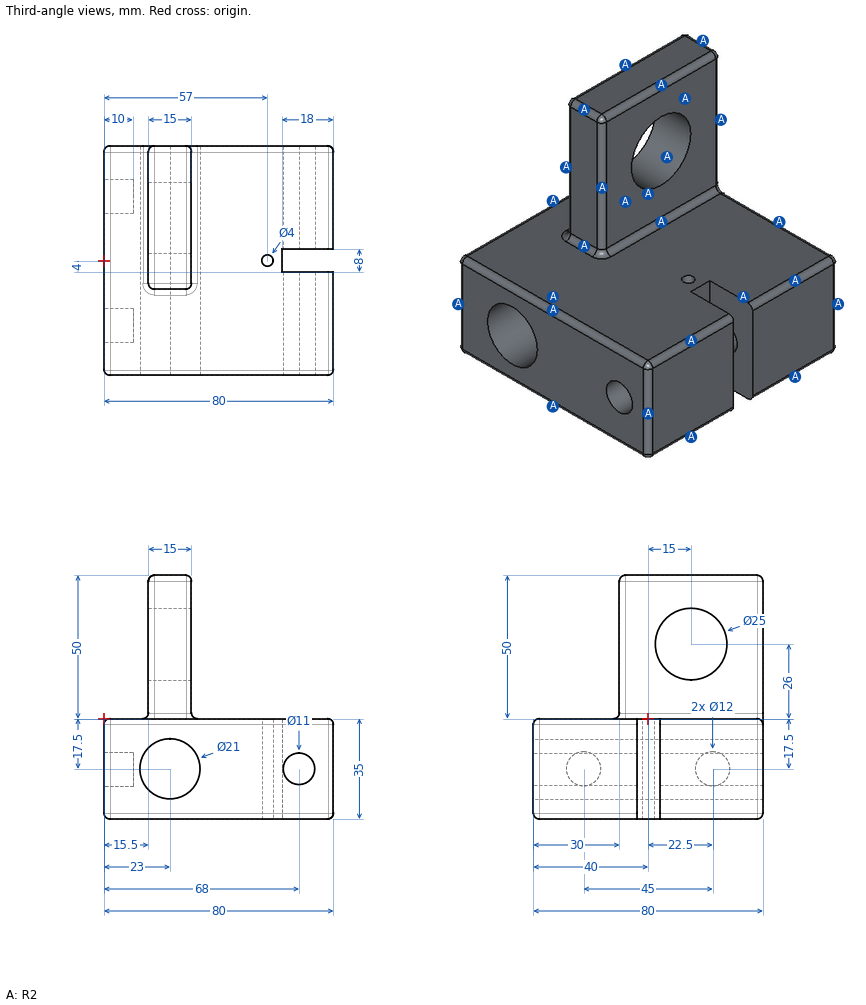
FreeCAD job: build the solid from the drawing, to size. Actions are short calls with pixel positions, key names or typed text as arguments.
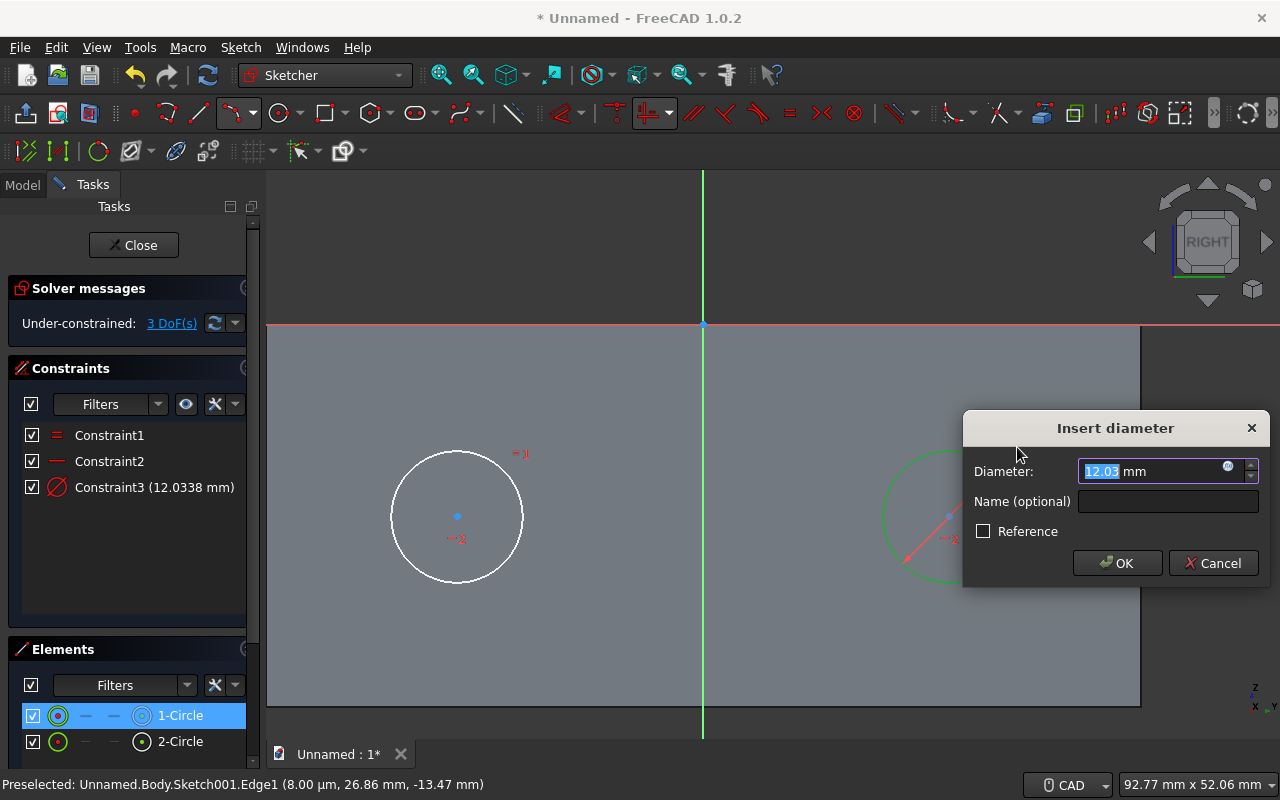
text(12)
key(Return)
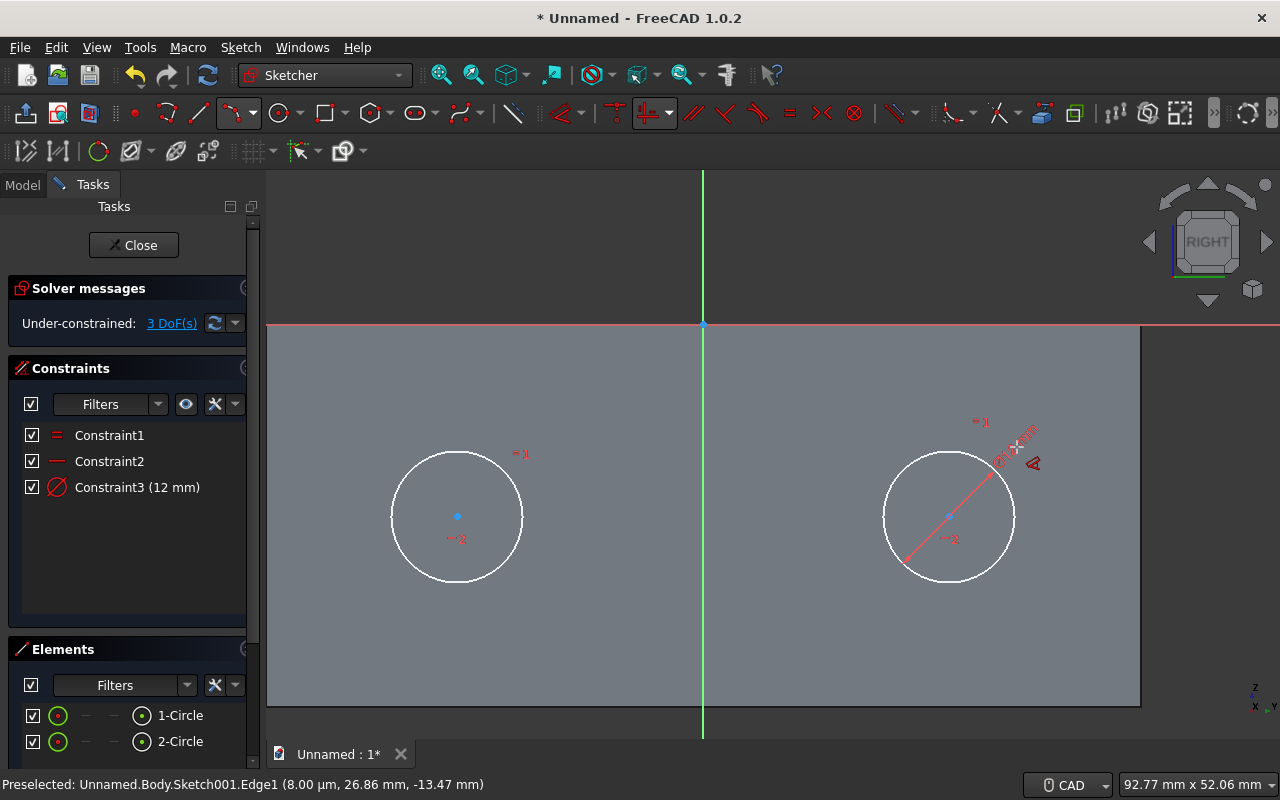
click(949, 517)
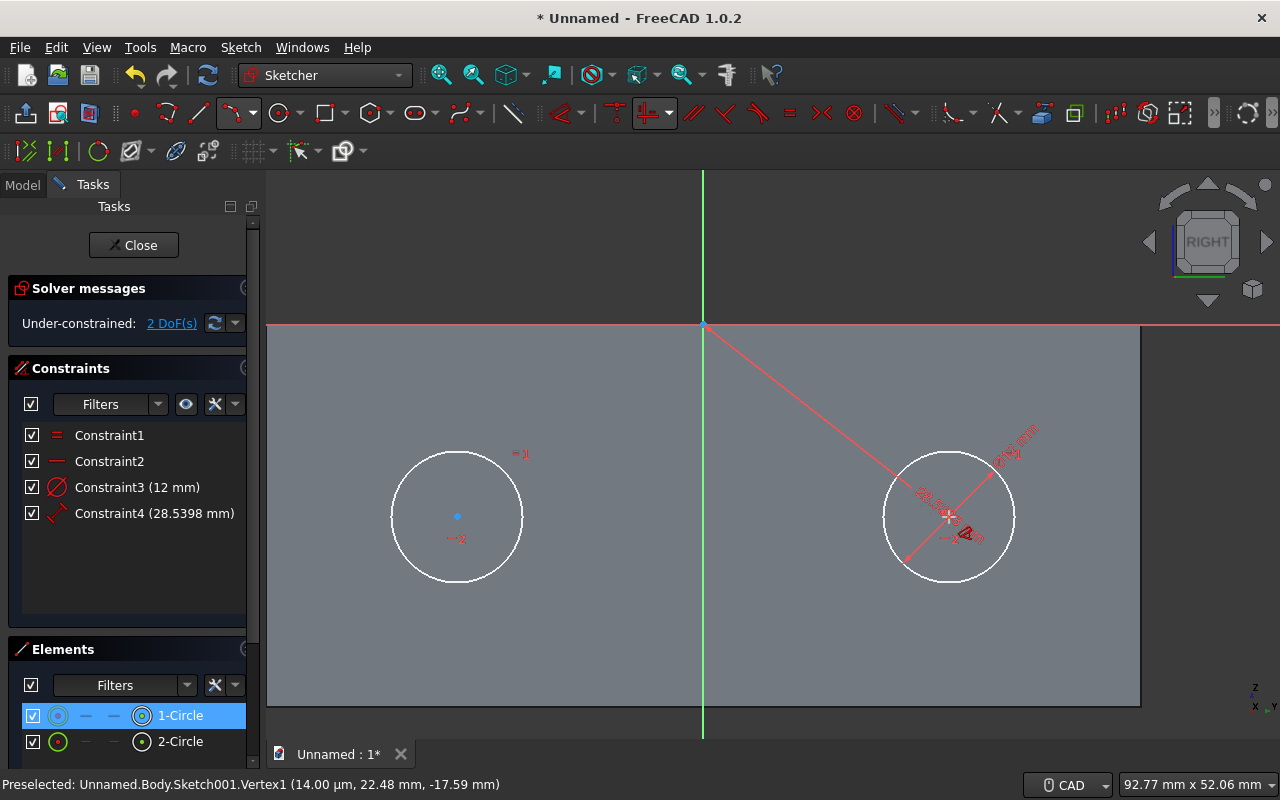
click(457, 517)
click(590, 551)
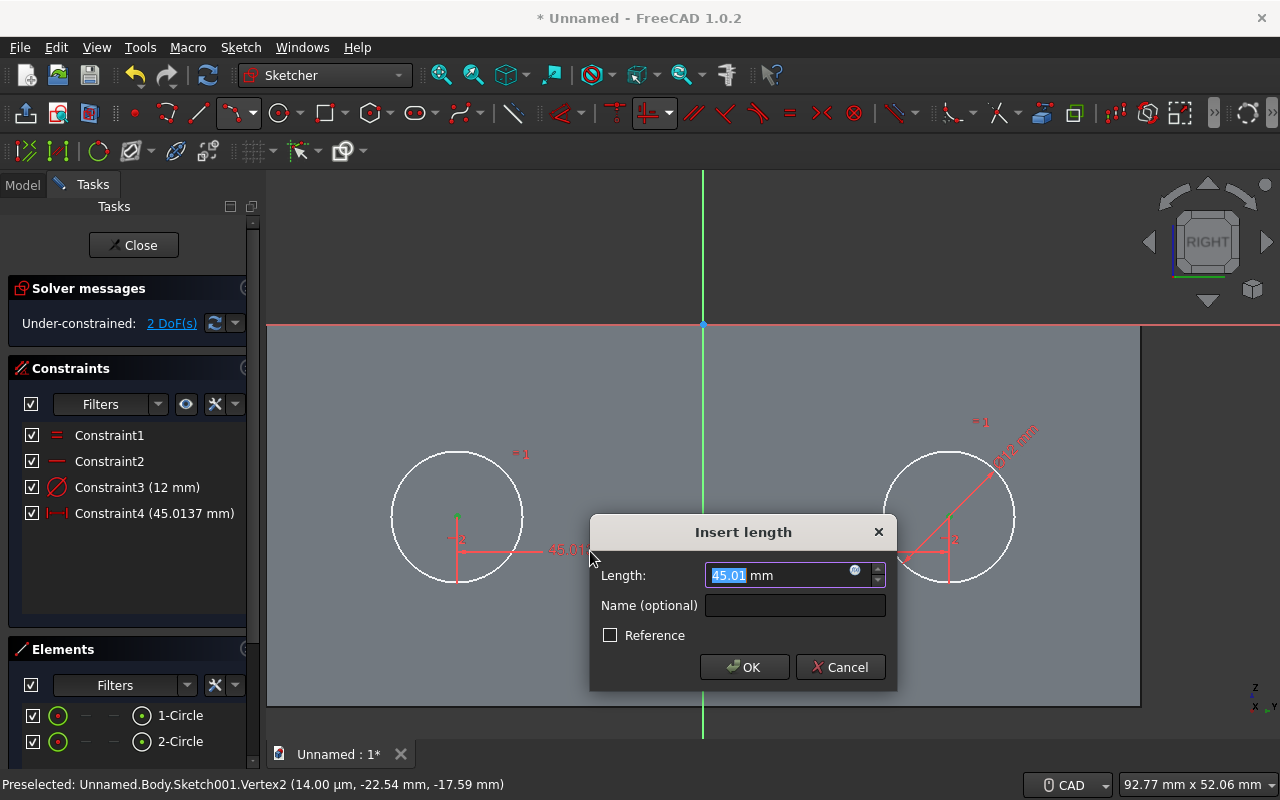
text(45)
key(Return)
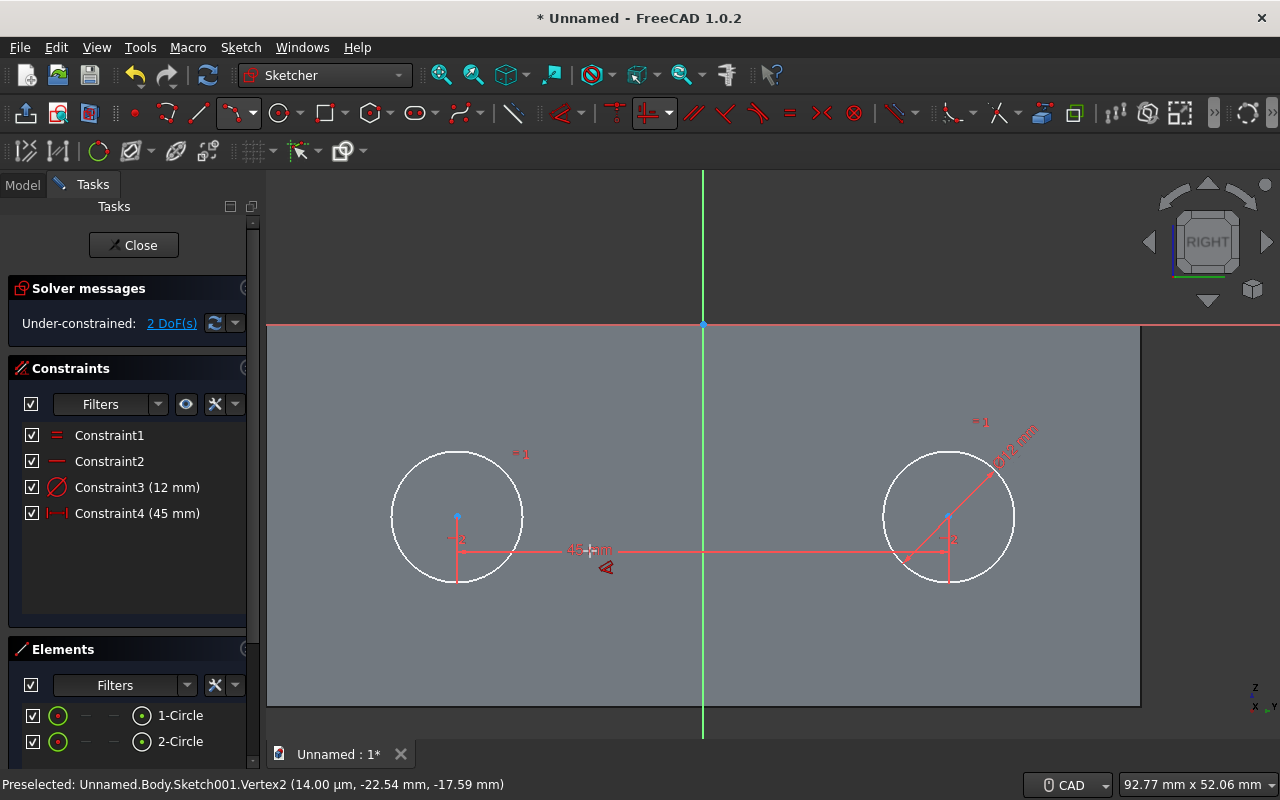
click(949, 517)
click(826, 291)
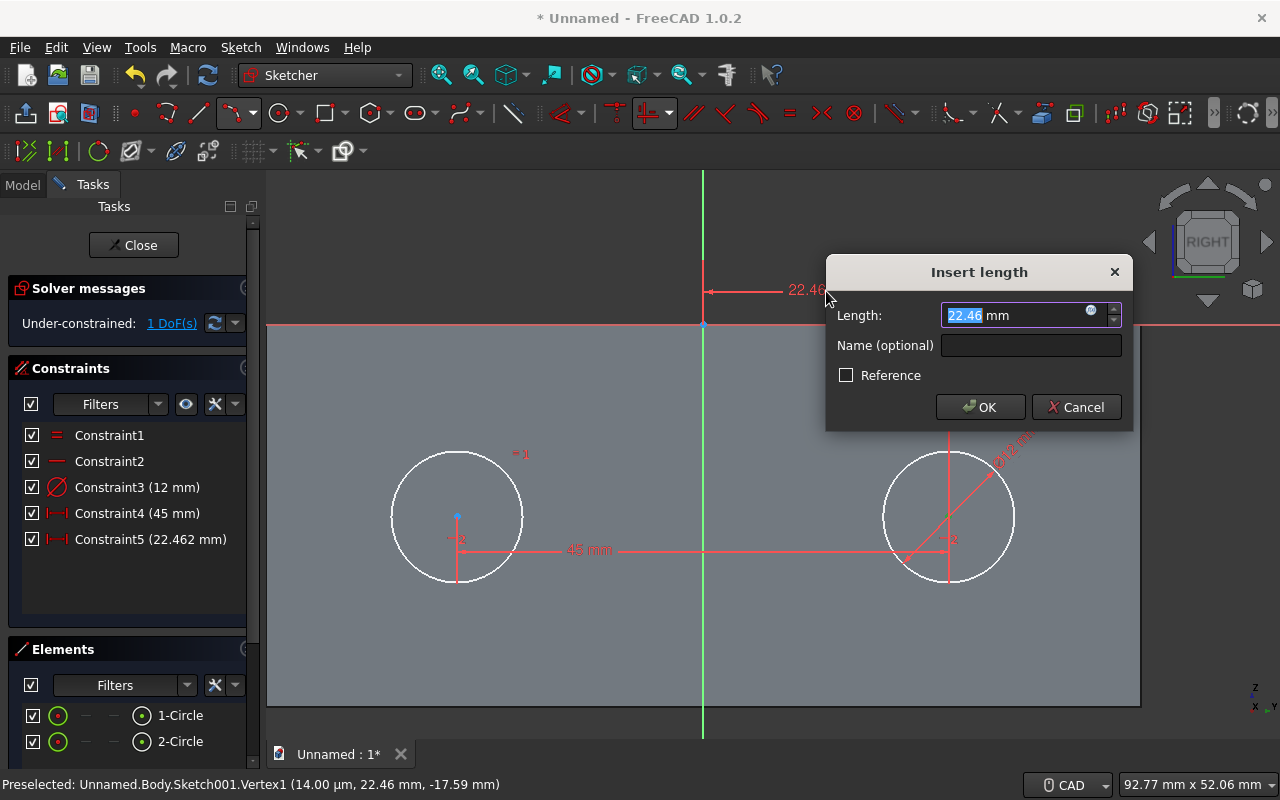
text(22.5)
key(Return)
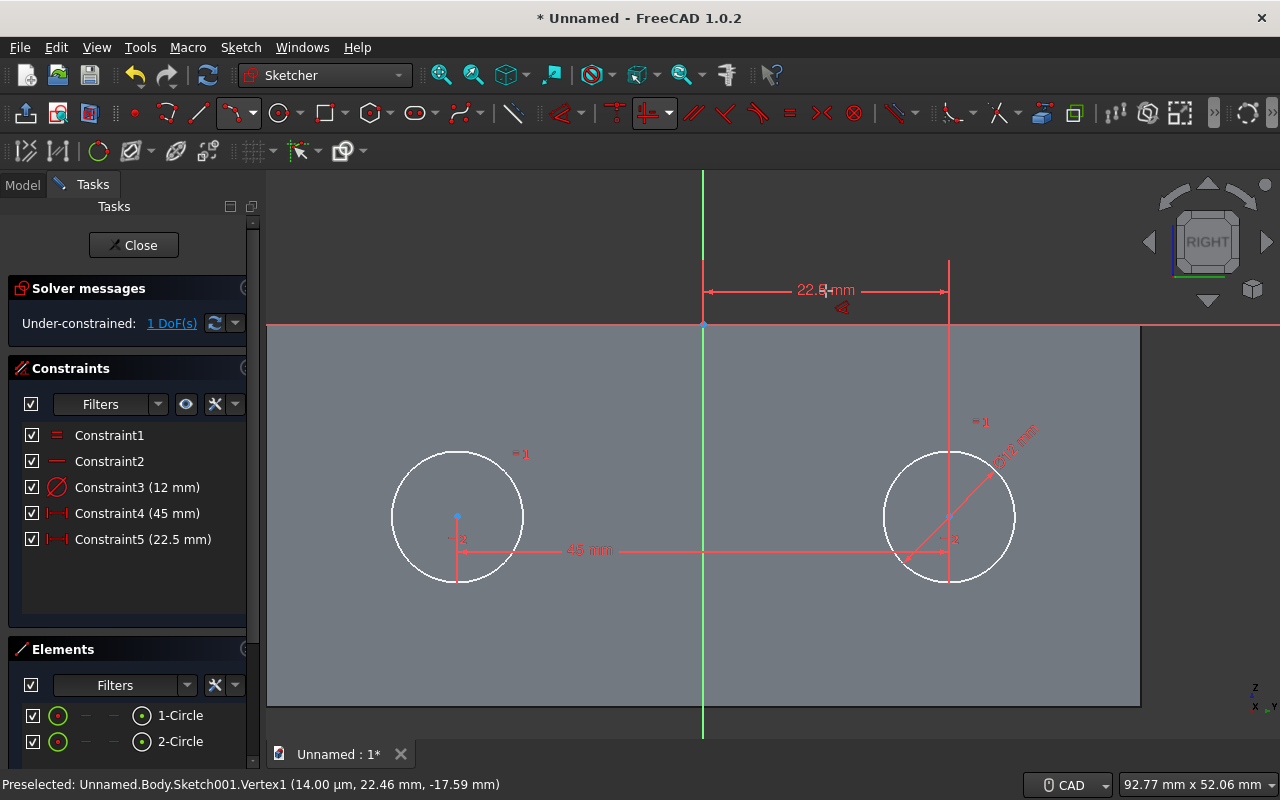
click(949, 517)
click(983, 421)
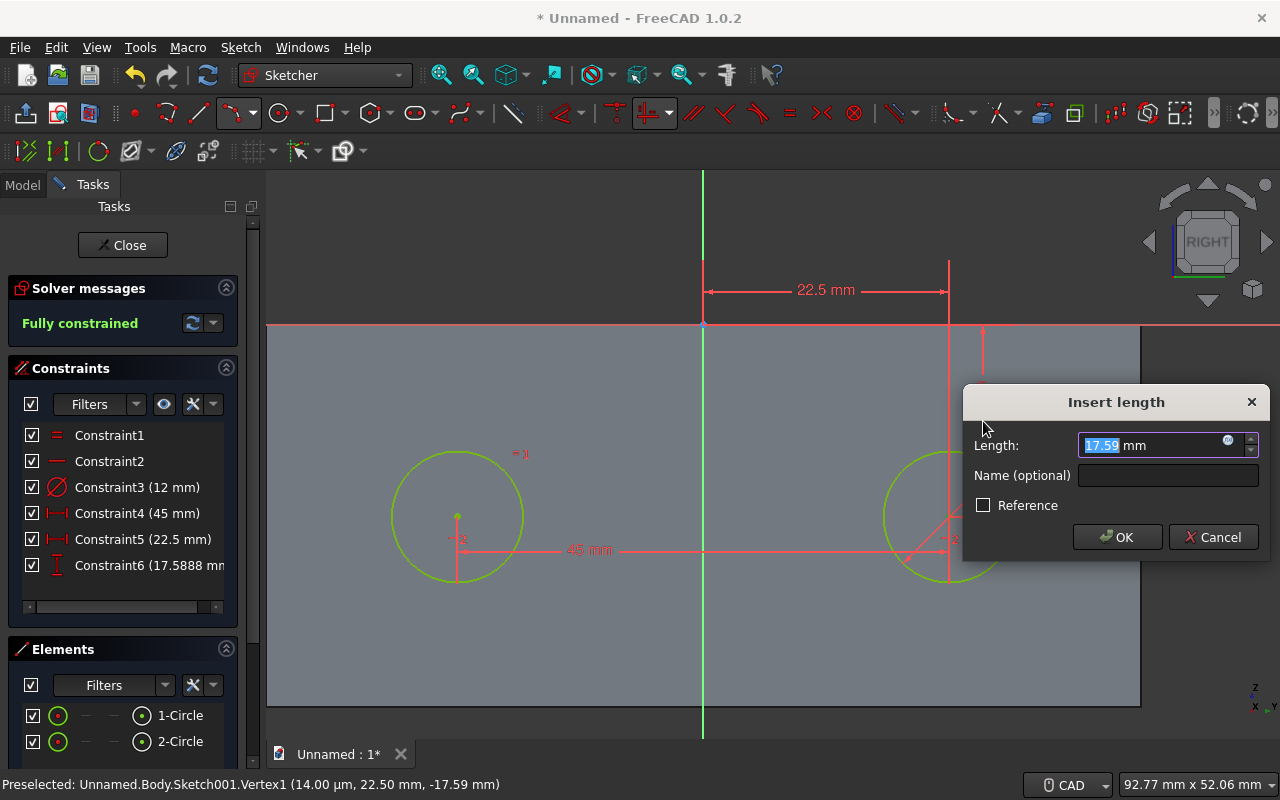
text(17.5)
key(Return)
key(Escape)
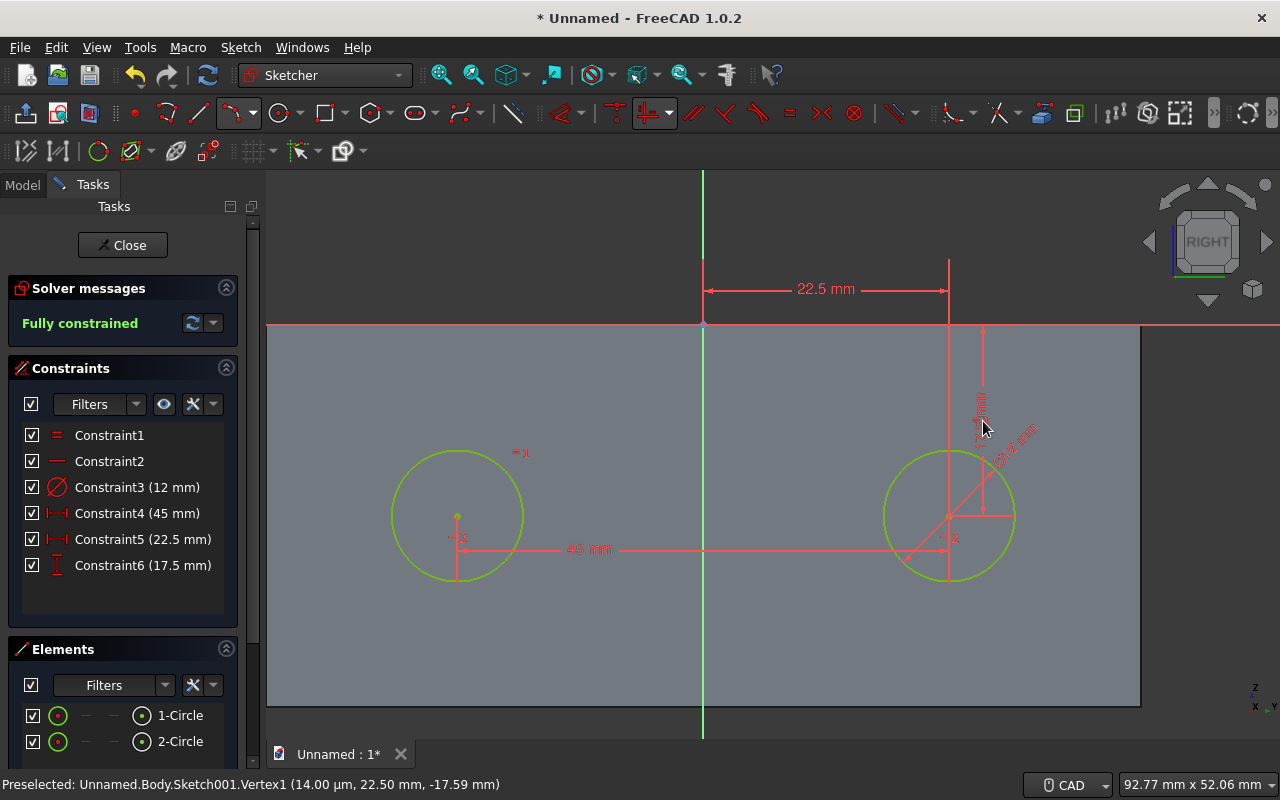
click(123, 245)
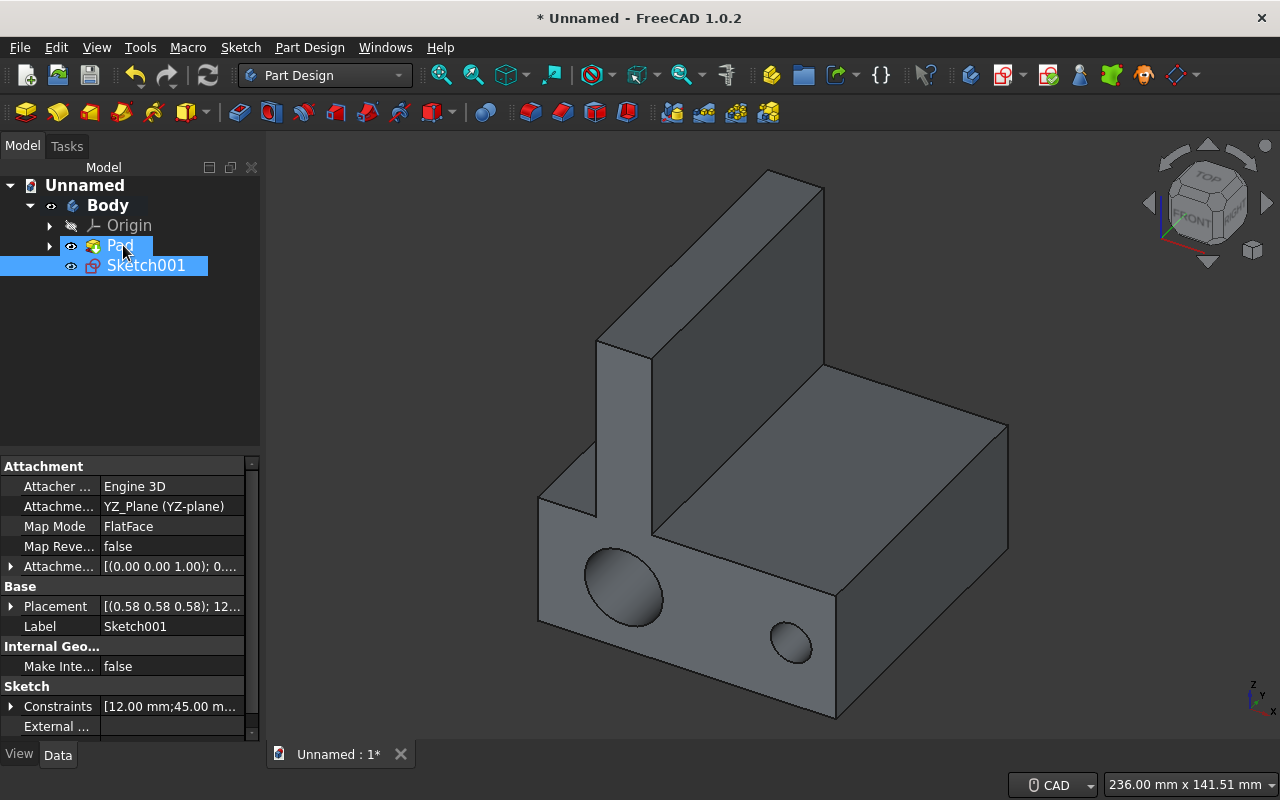
click(240, 112)